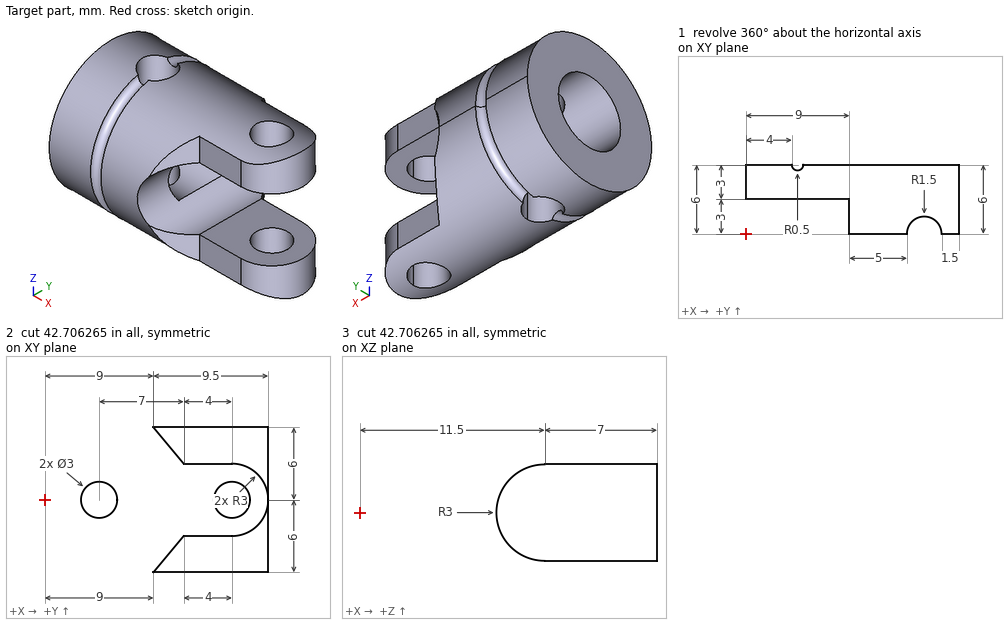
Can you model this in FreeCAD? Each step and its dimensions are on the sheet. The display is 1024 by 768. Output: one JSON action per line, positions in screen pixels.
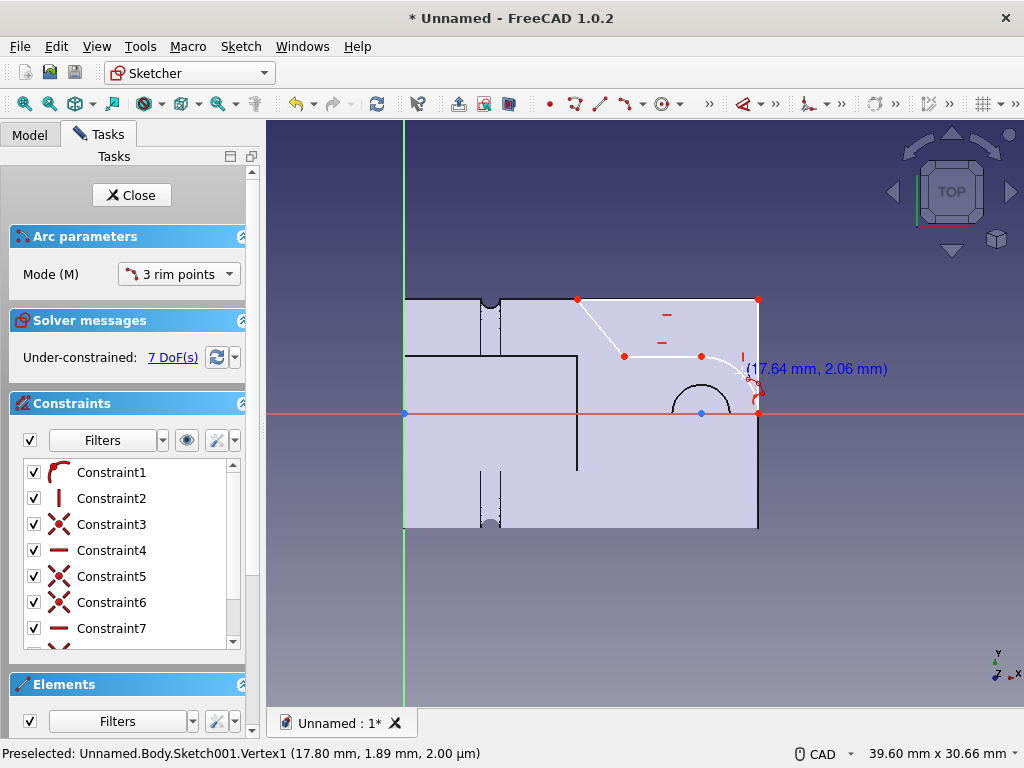
{"action": "key", "text": "g m"}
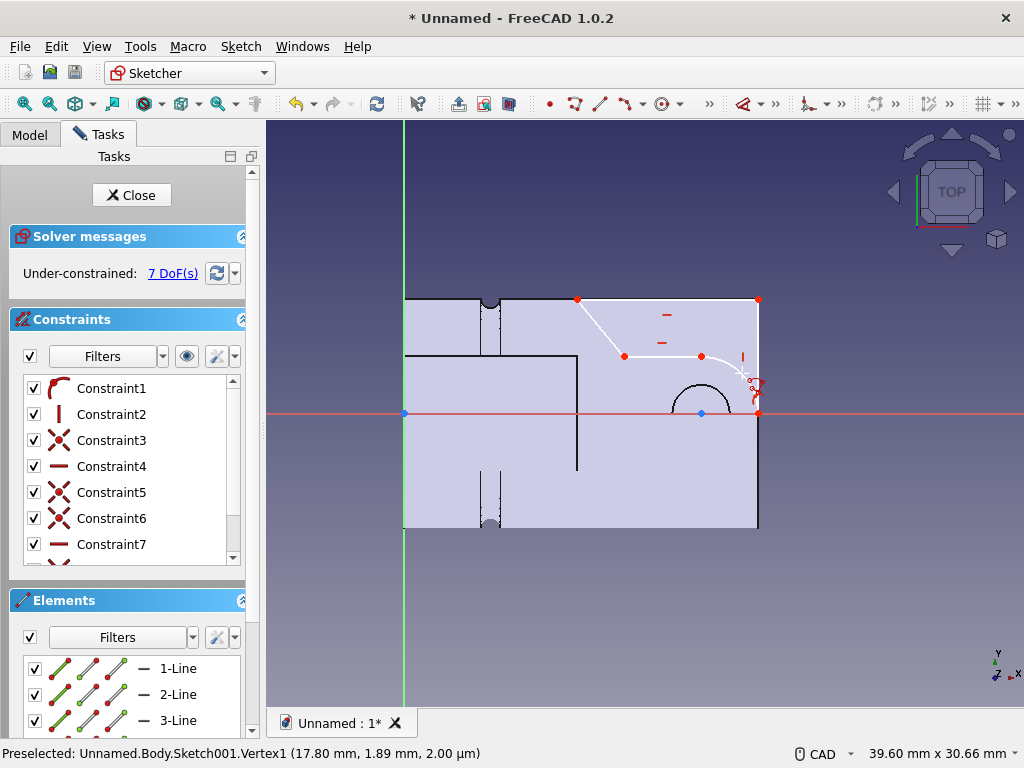
{"action": "left_click", "coordinate": [701, 471]}
{"action": "left_click", "coordinate": [624, 471]}
{"action": "left_click", "coordinate": [577, 528]}
{"action": "left_click", "coordinate": [758, 528]}
{"action": "left_click", "coordinate": [758, 414]}
{"action": "right_click", "coordinate": [758, 528]}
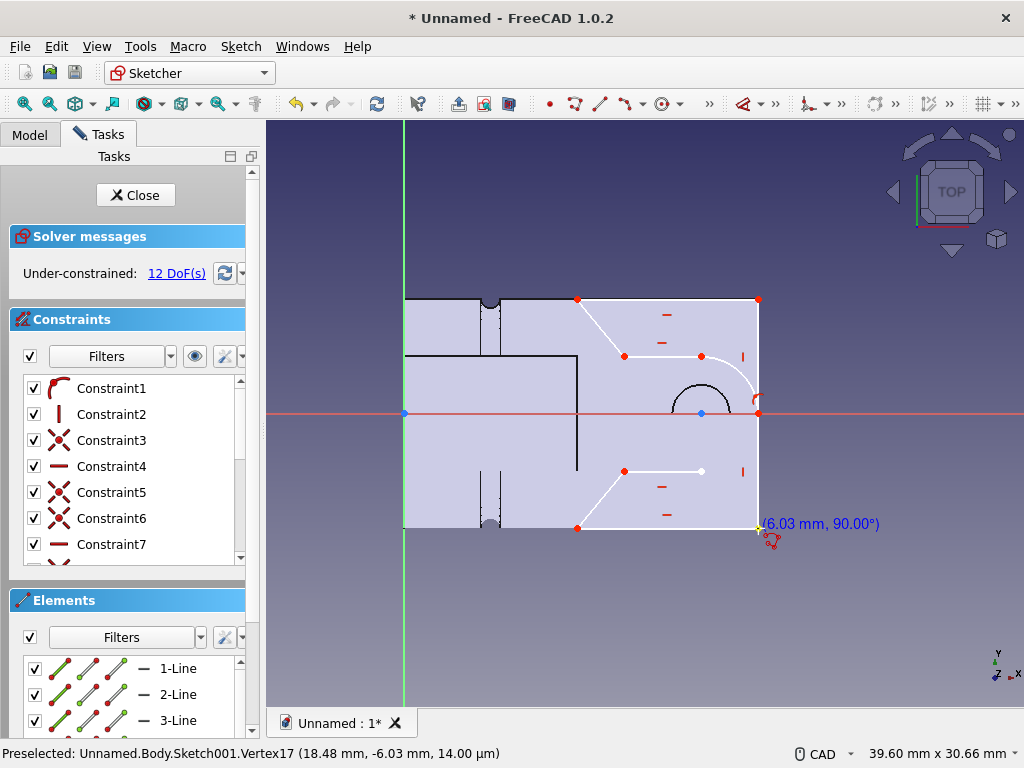
{"action": "left_click", "coordinate": [624, 104]}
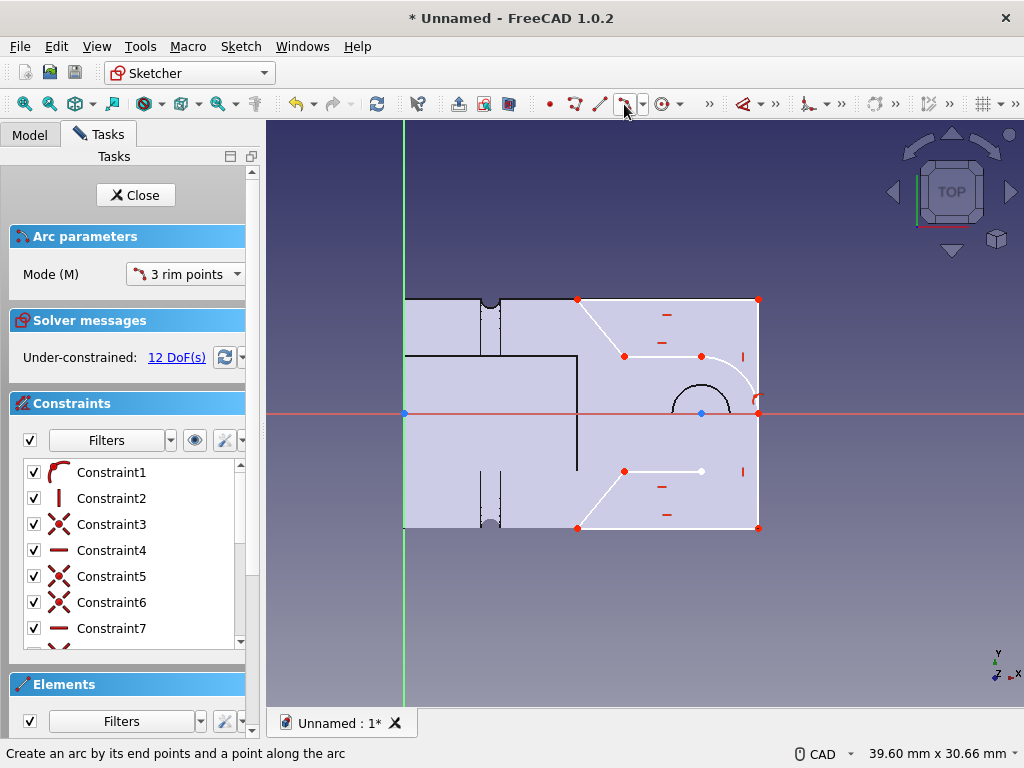
{"action": "left_click", "coordinate": [758, 414]}
{"action": "left_click", "coordinate": [701, 472]}
{"action": "left_click", "coordinate": [742, 454]}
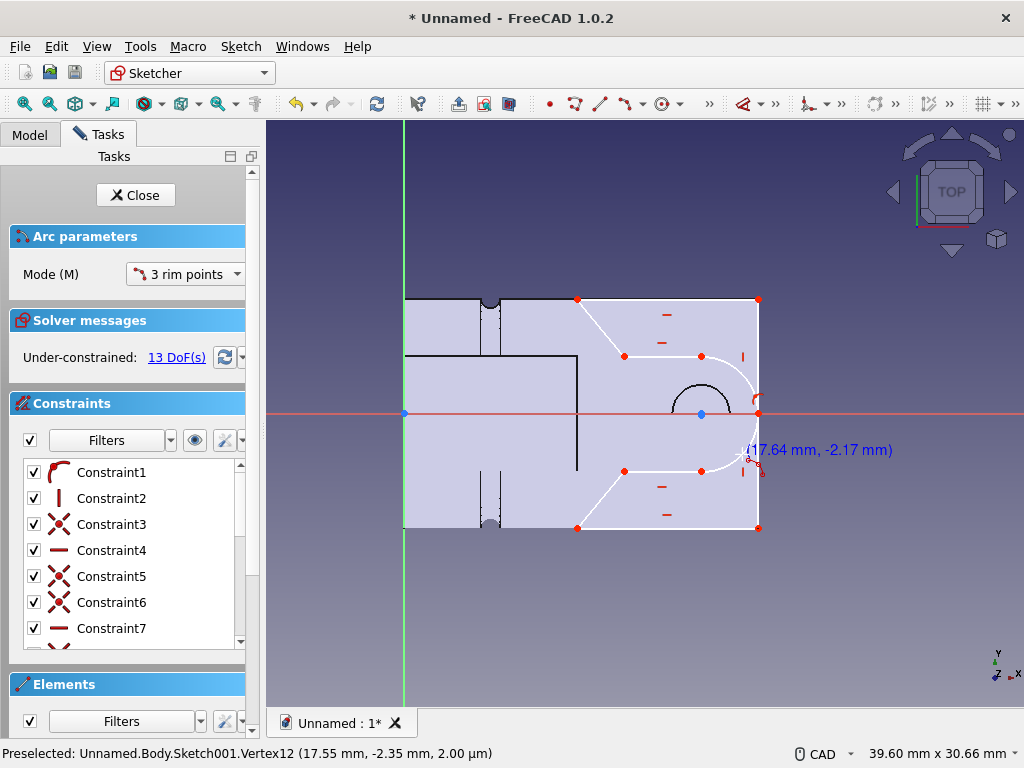
{"action": "left_click", "coordinate": [662, 104]}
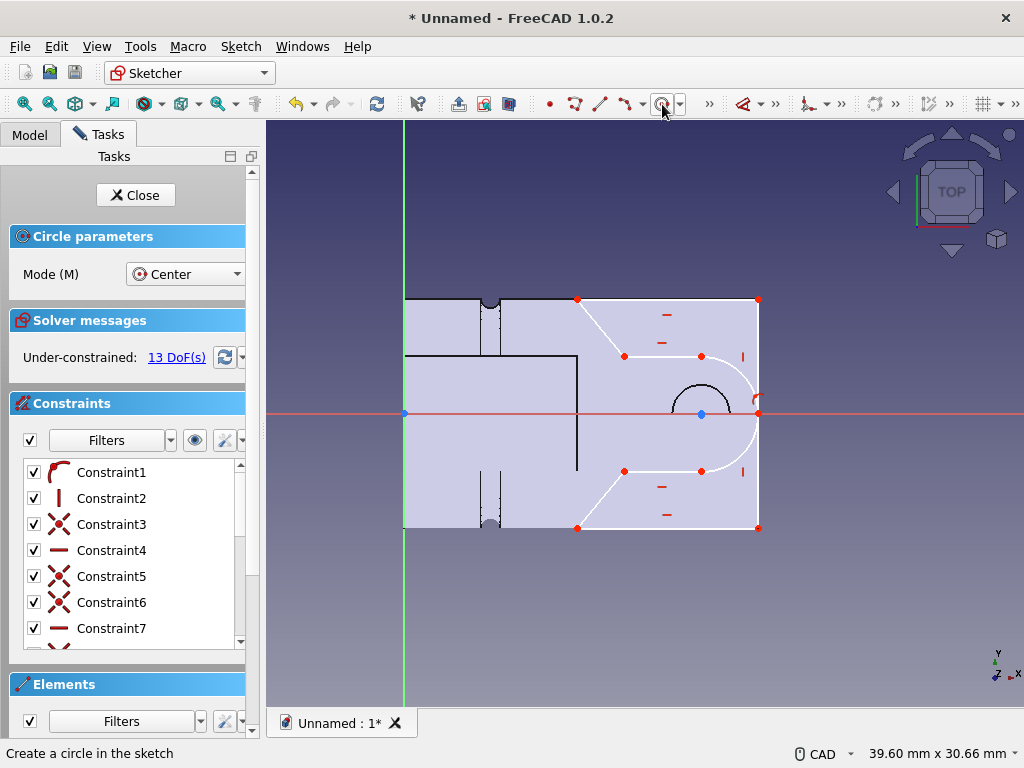
{"action": "left_click", "coordinate": [701, 414]}
{"action": "left_click", "coordinate": [721, 393]}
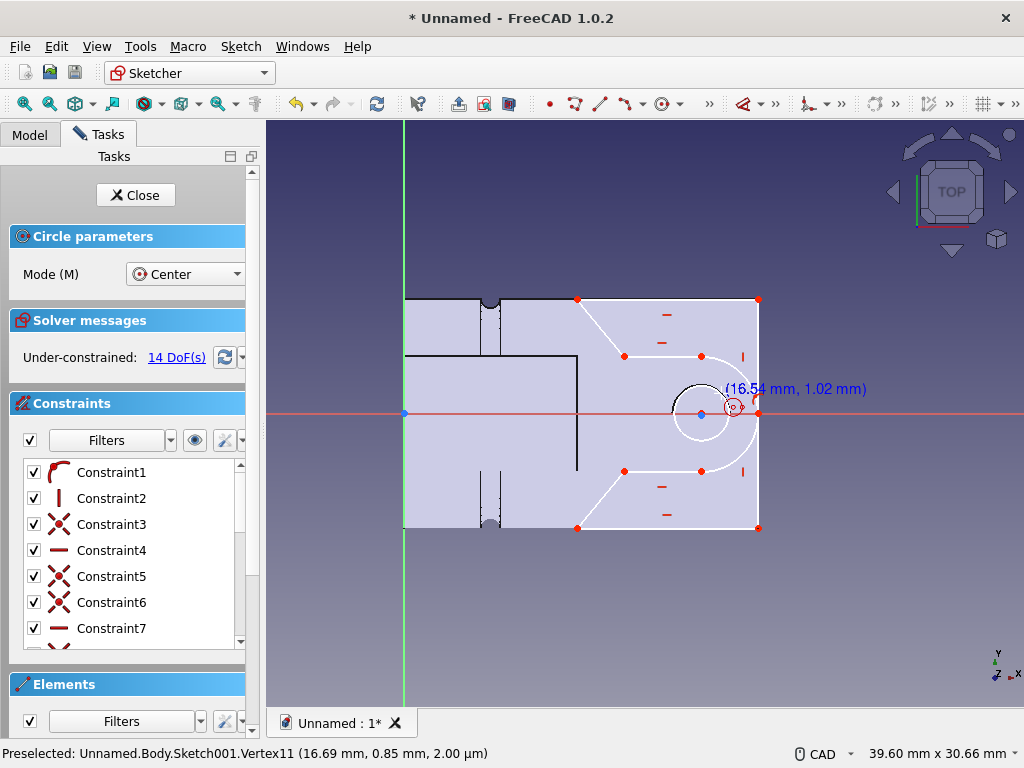
{"action": "left_click", "coordinate": [490, 414]}
{"action": "left_click", "coordinate": [511, 393]}
{"action": "key", "text": "Escape"}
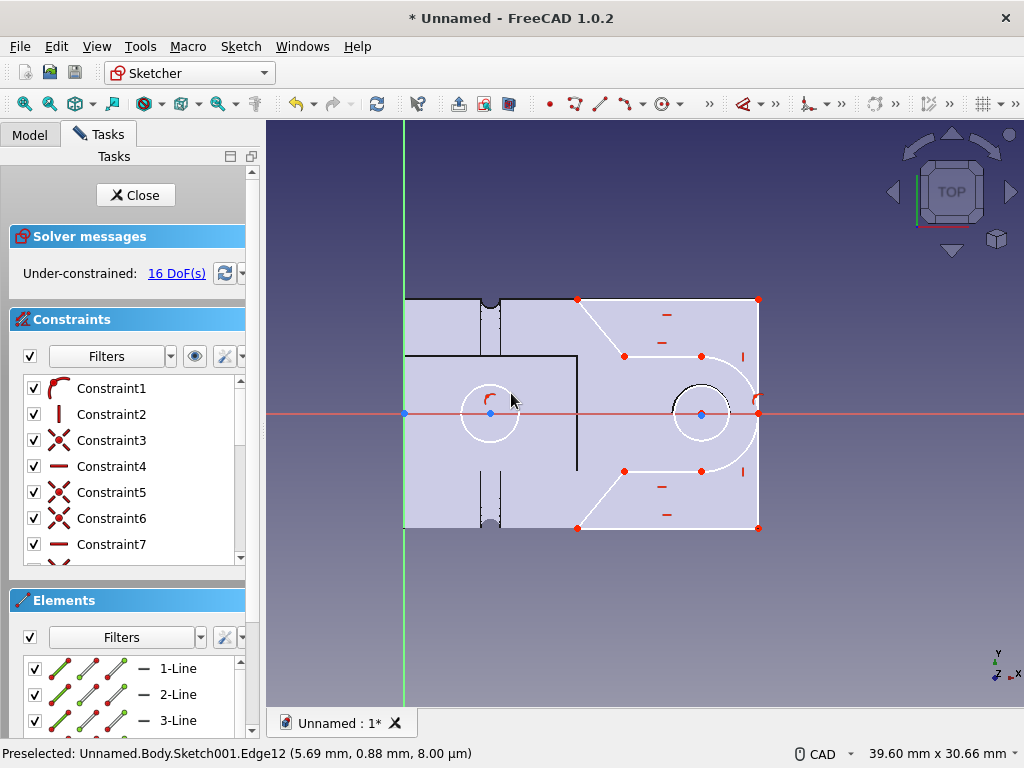
{"action": "scroll", "coordinate": [758, 379], "scroll_direction": "up", "scroll_amount": 2}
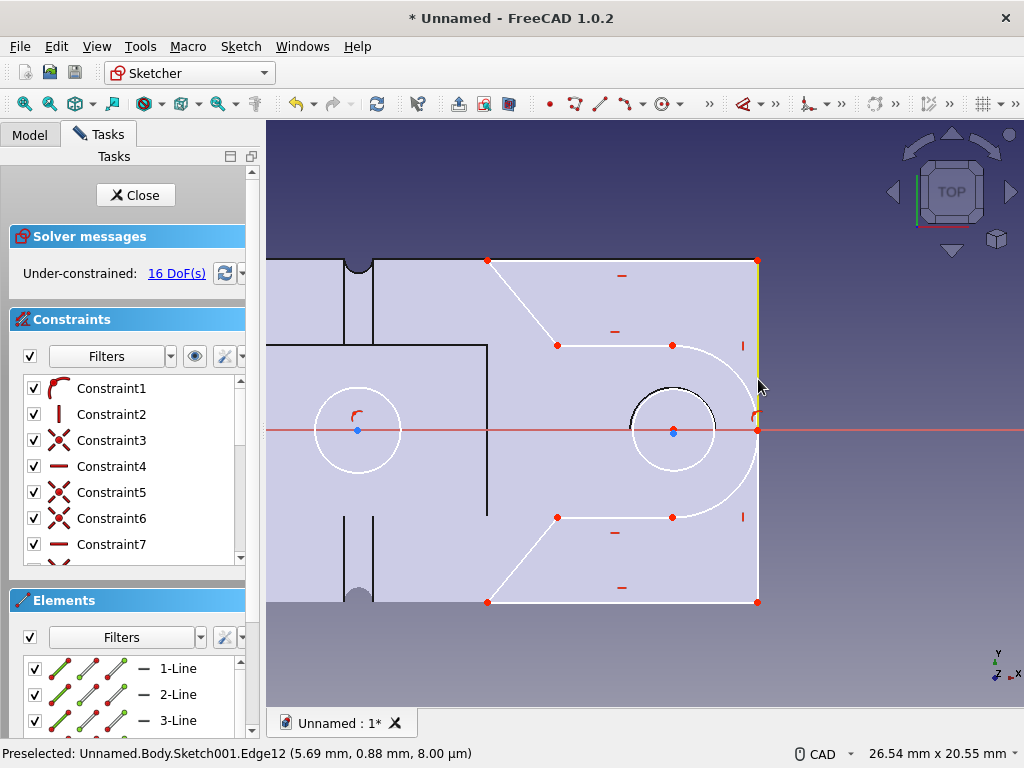
{"action": "left_click", "coordinate": [758, 379]}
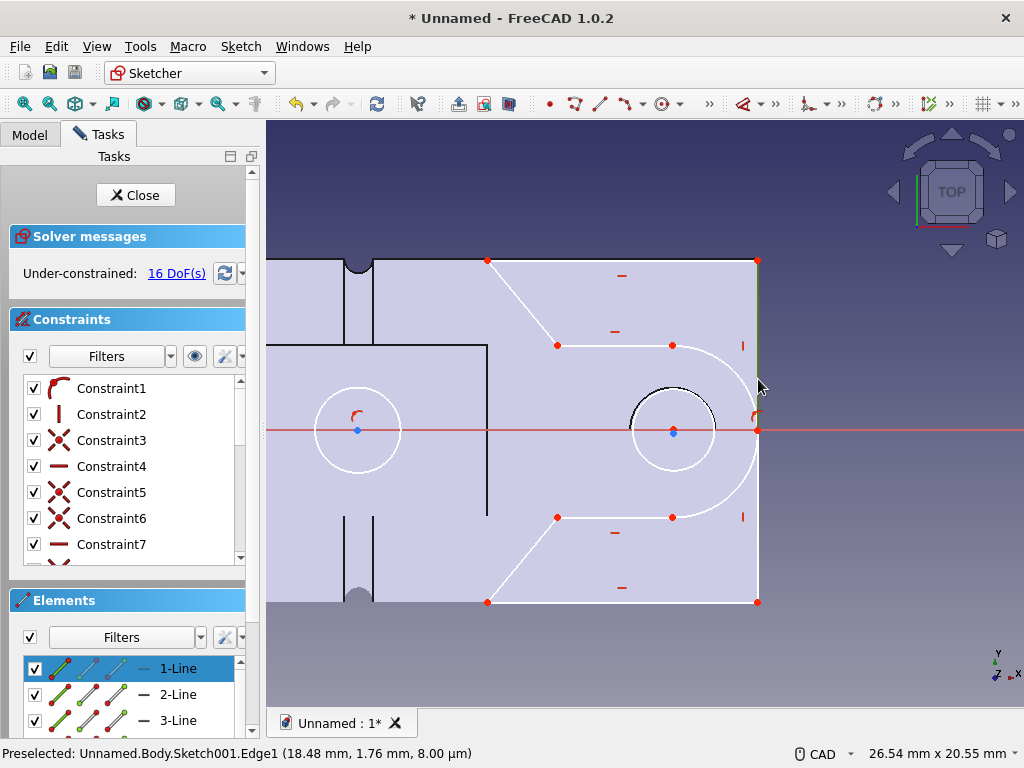
{"action": "scroll", "coordinate": [748, 392], "scroll_direction": "up", "scroll_amount": 3}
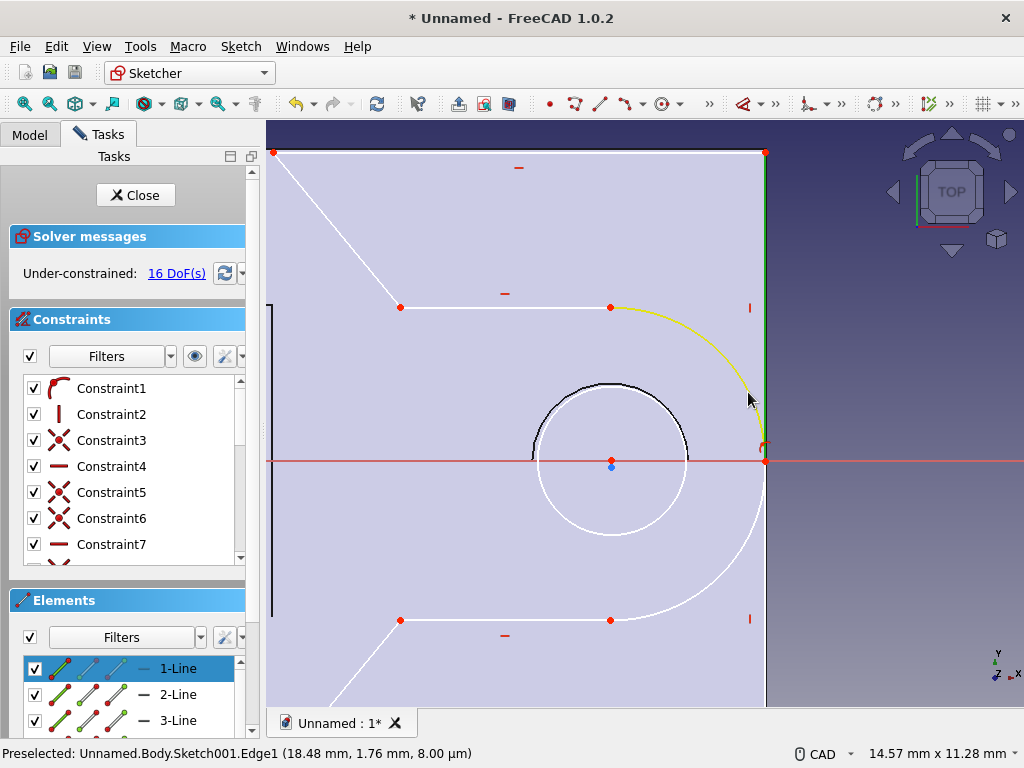
{"action": "left_click", "coordinate": [748, 391]}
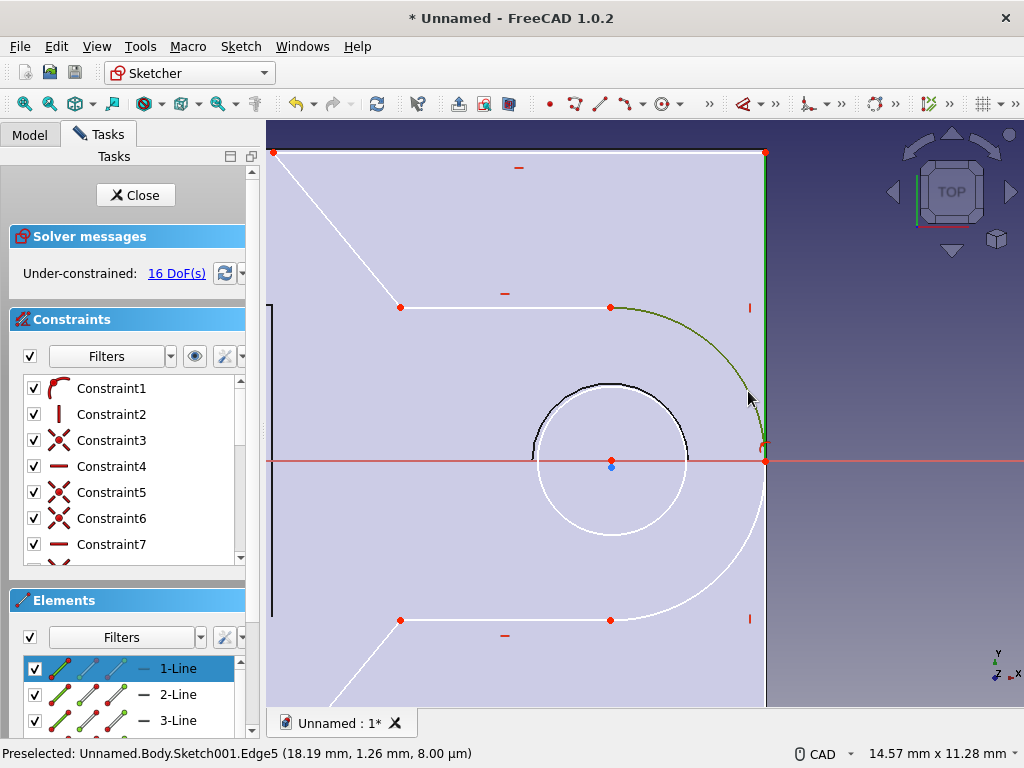
{"action": "key", "text": "t"}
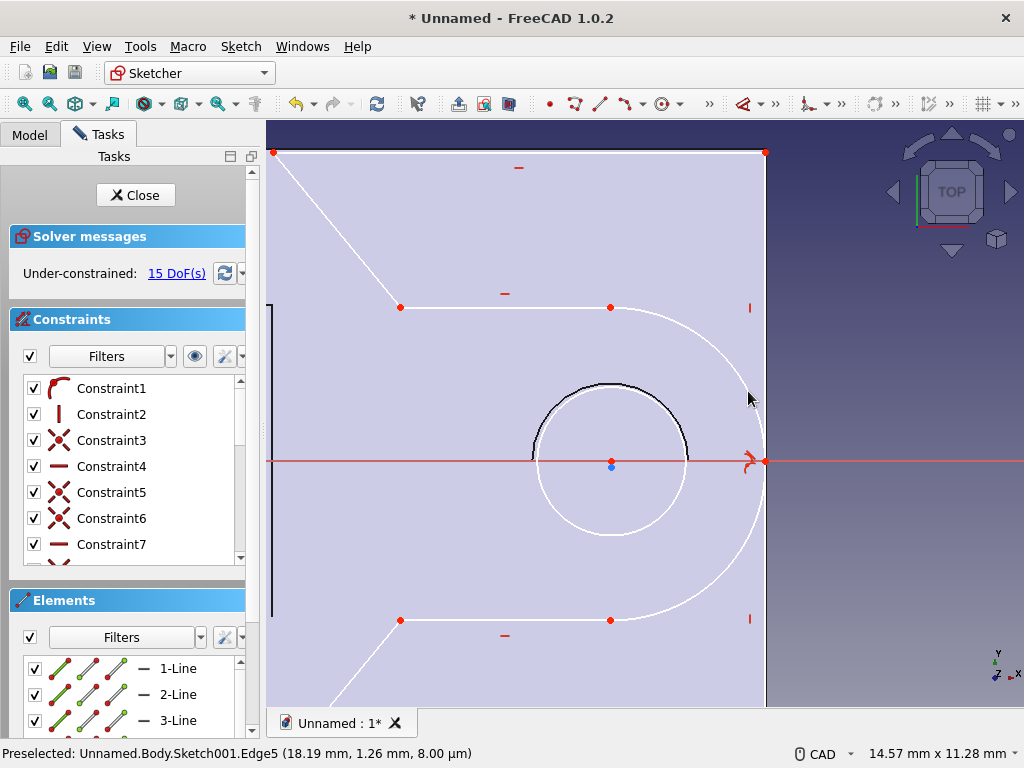
{"action": "left_click", "coordinate": [765, 369]}